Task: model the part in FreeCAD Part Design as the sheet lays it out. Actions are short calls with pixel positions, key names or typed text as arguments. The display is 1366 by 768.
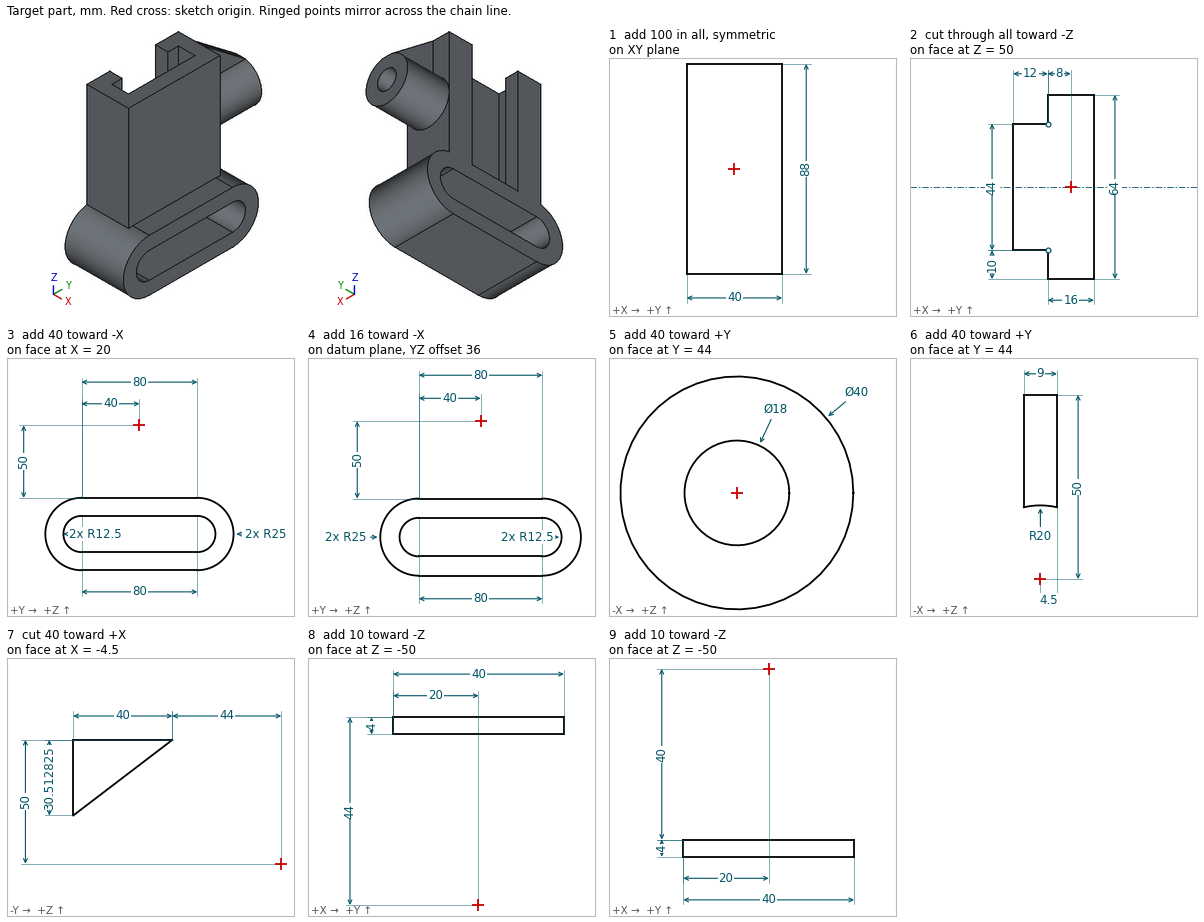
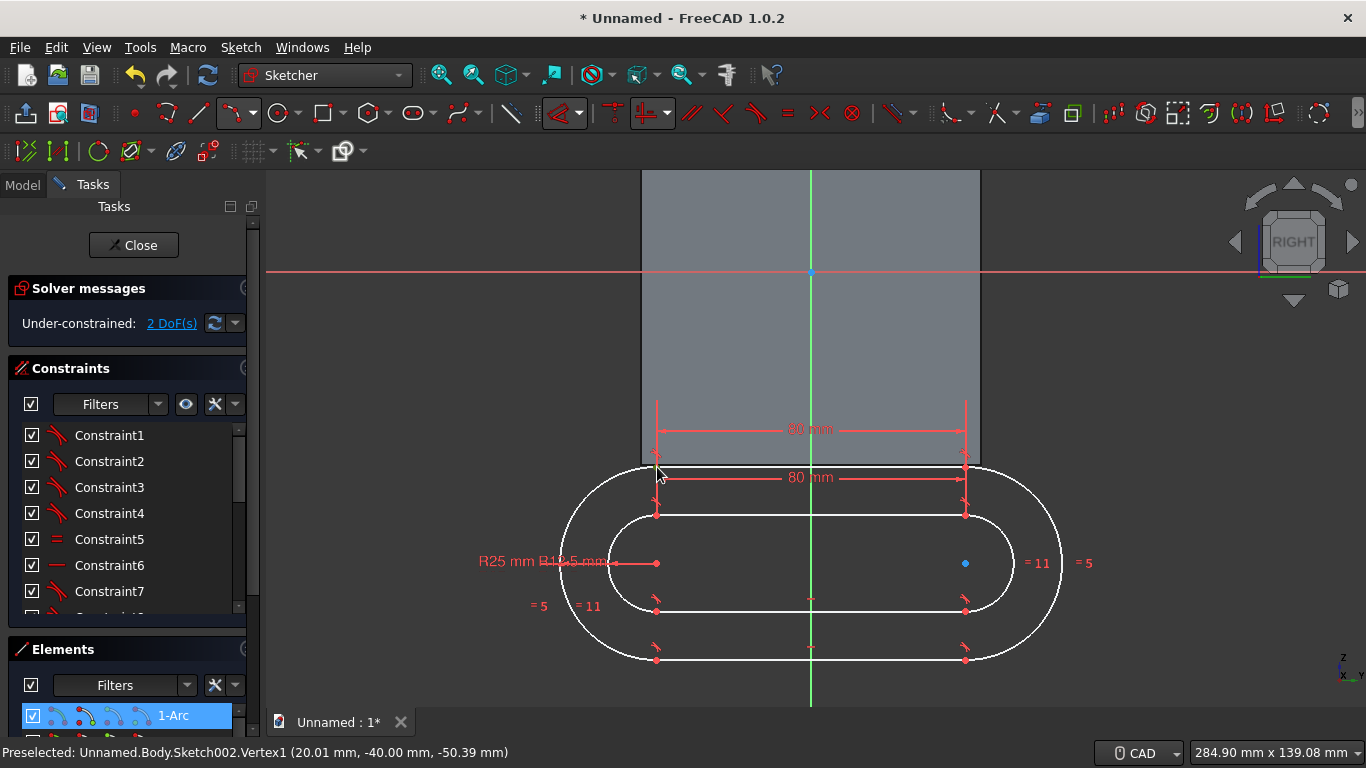
key(l)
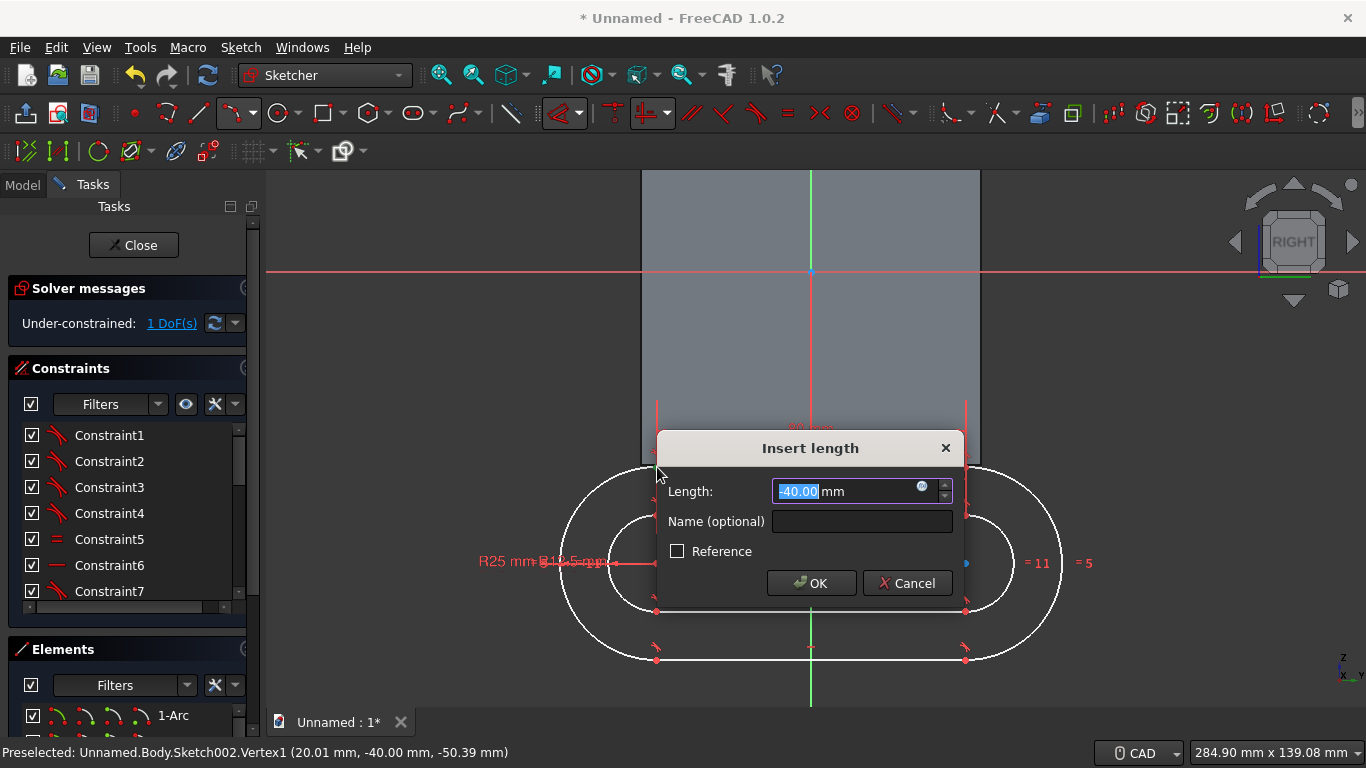
text(-40)
key(Return)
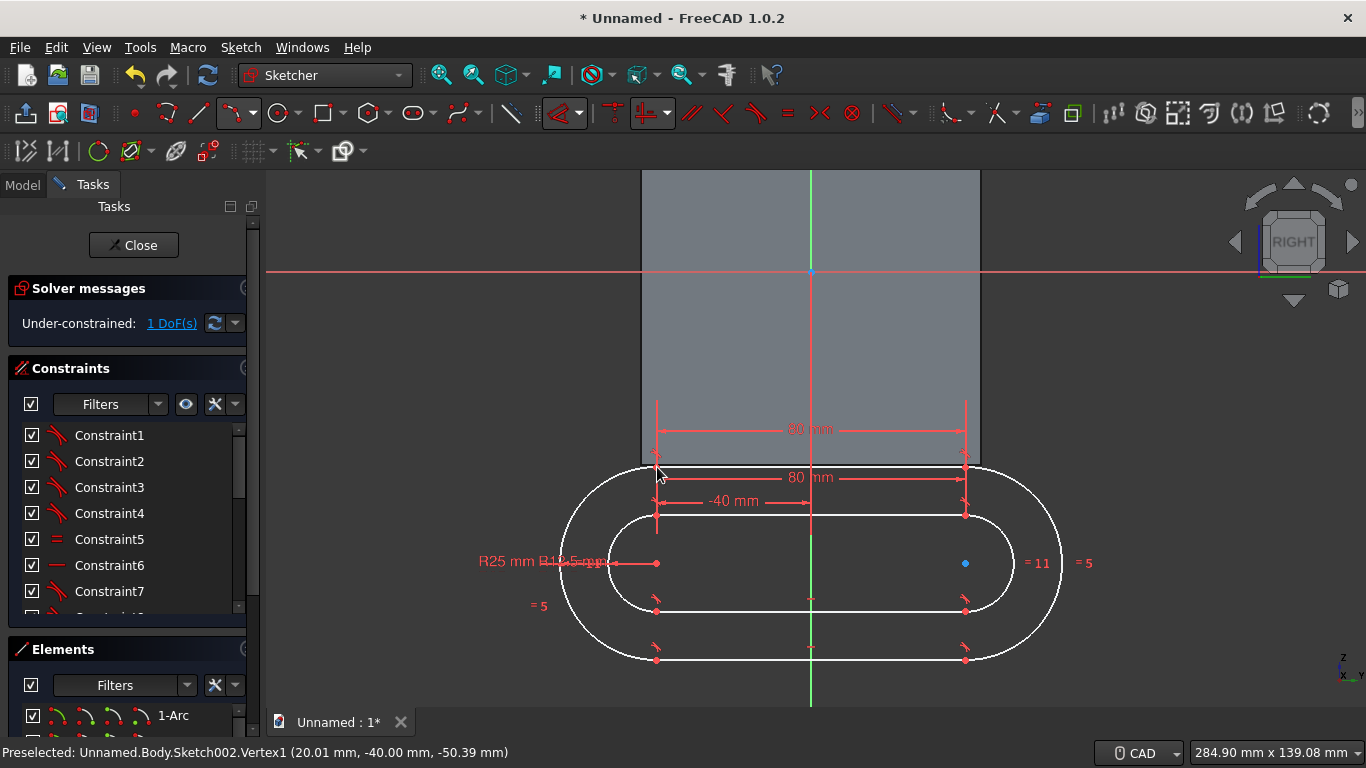
click(657, 467)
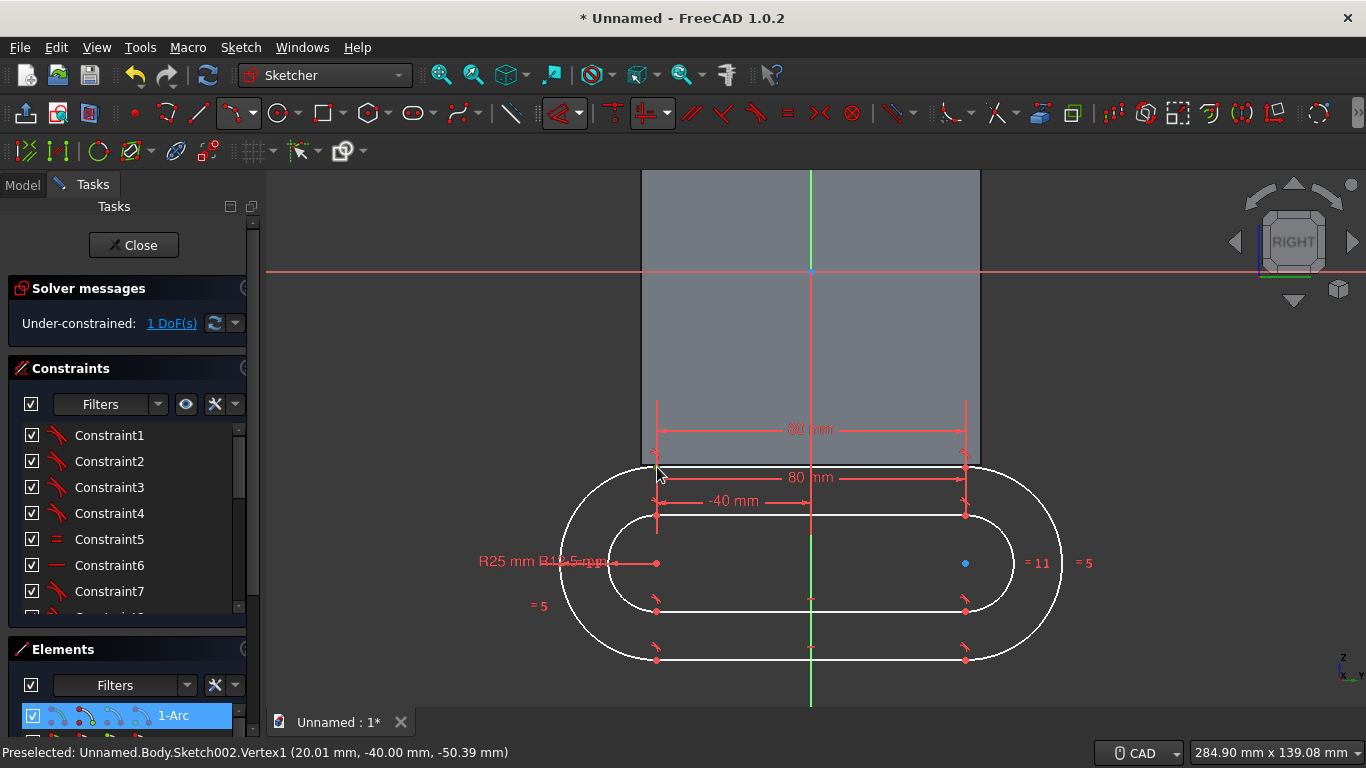
key(i)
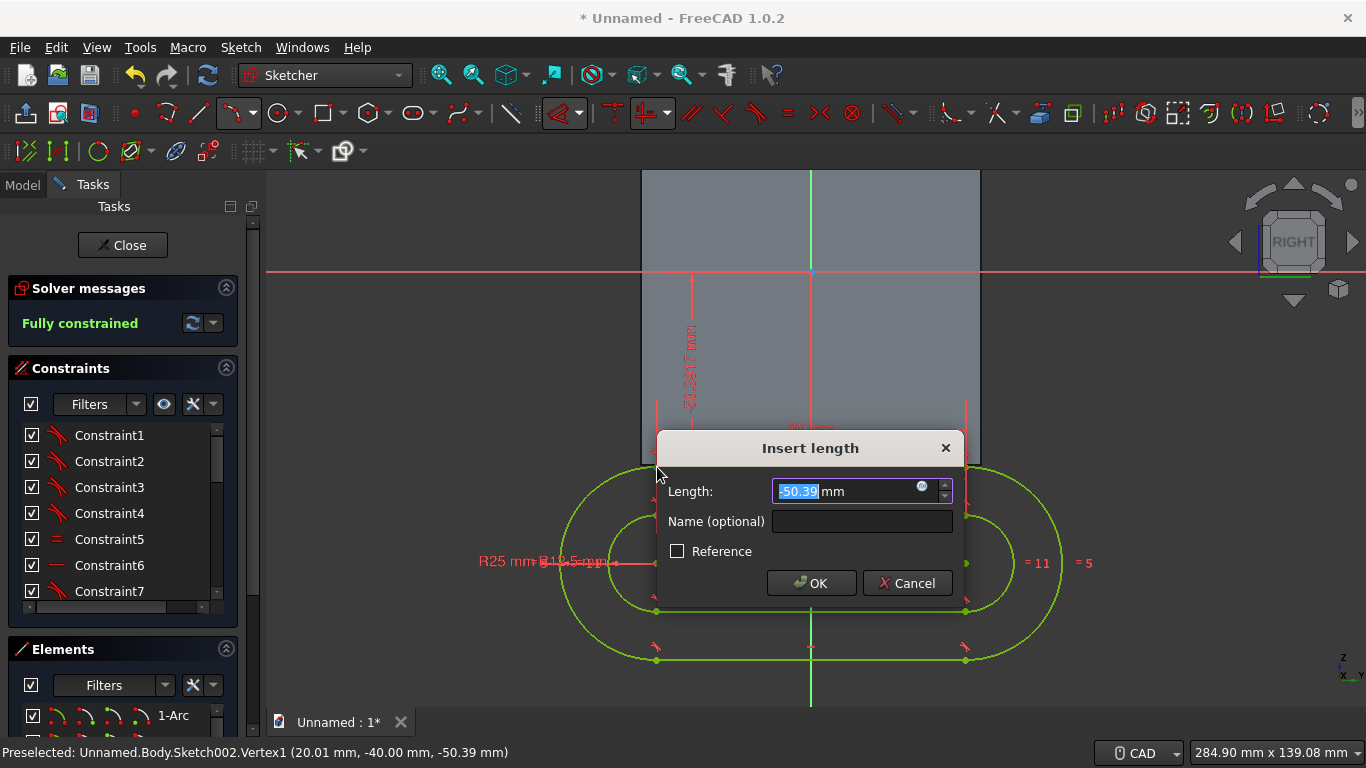
text(-50)
key(Return)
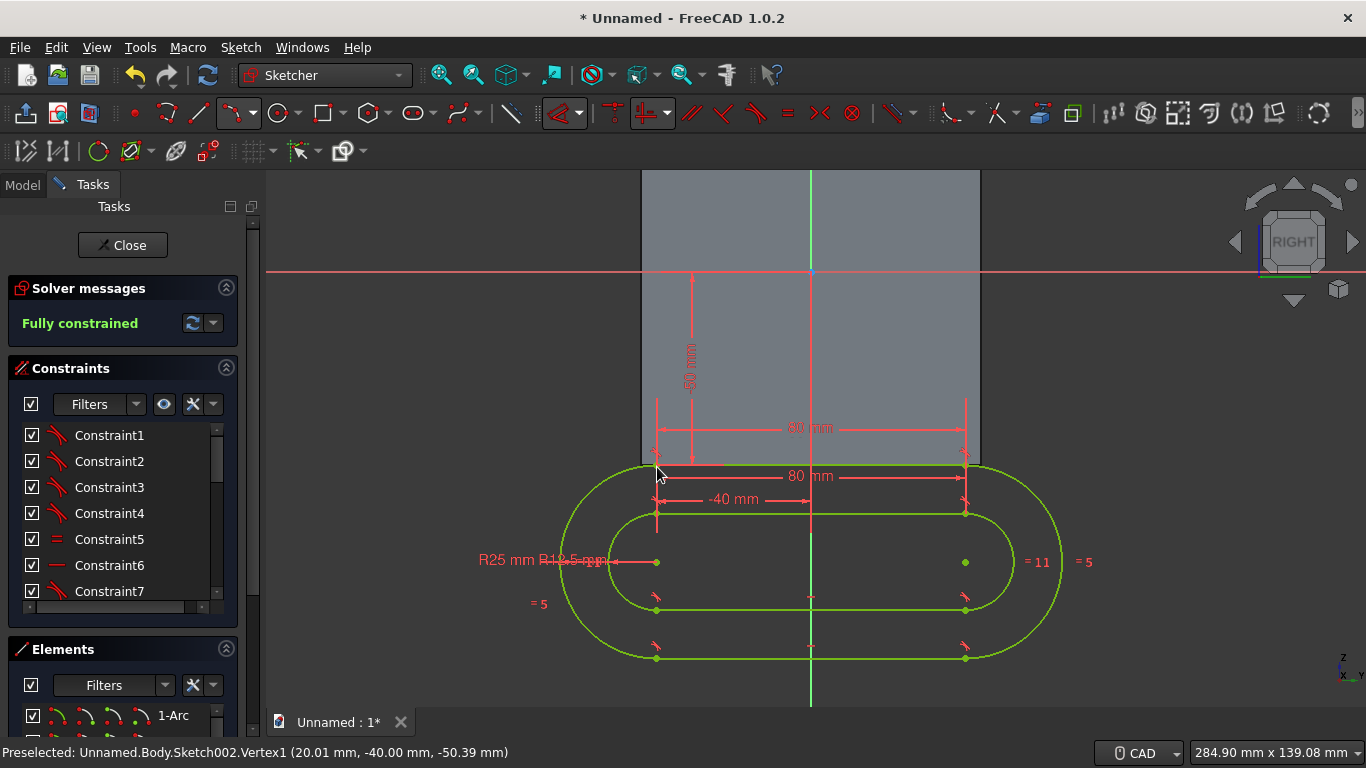
click(123, 245)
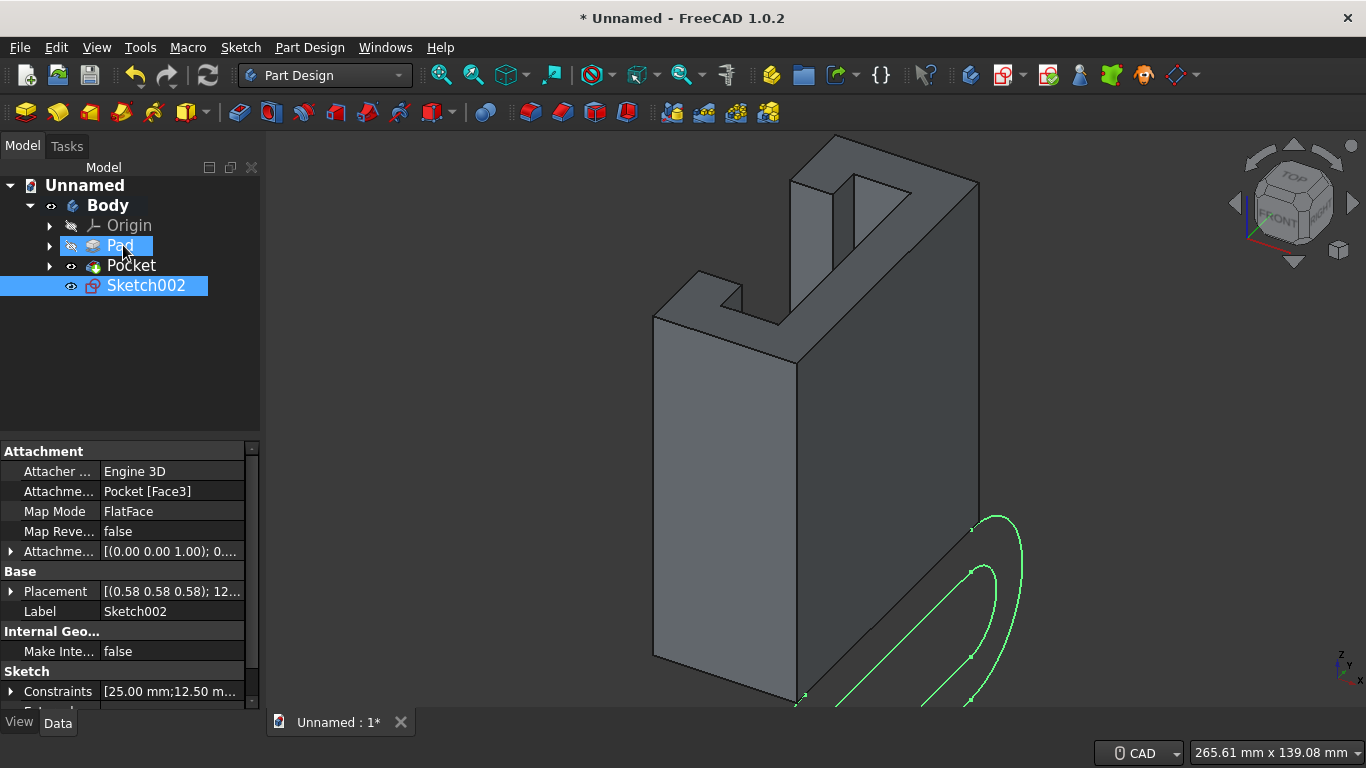
click(26, 112)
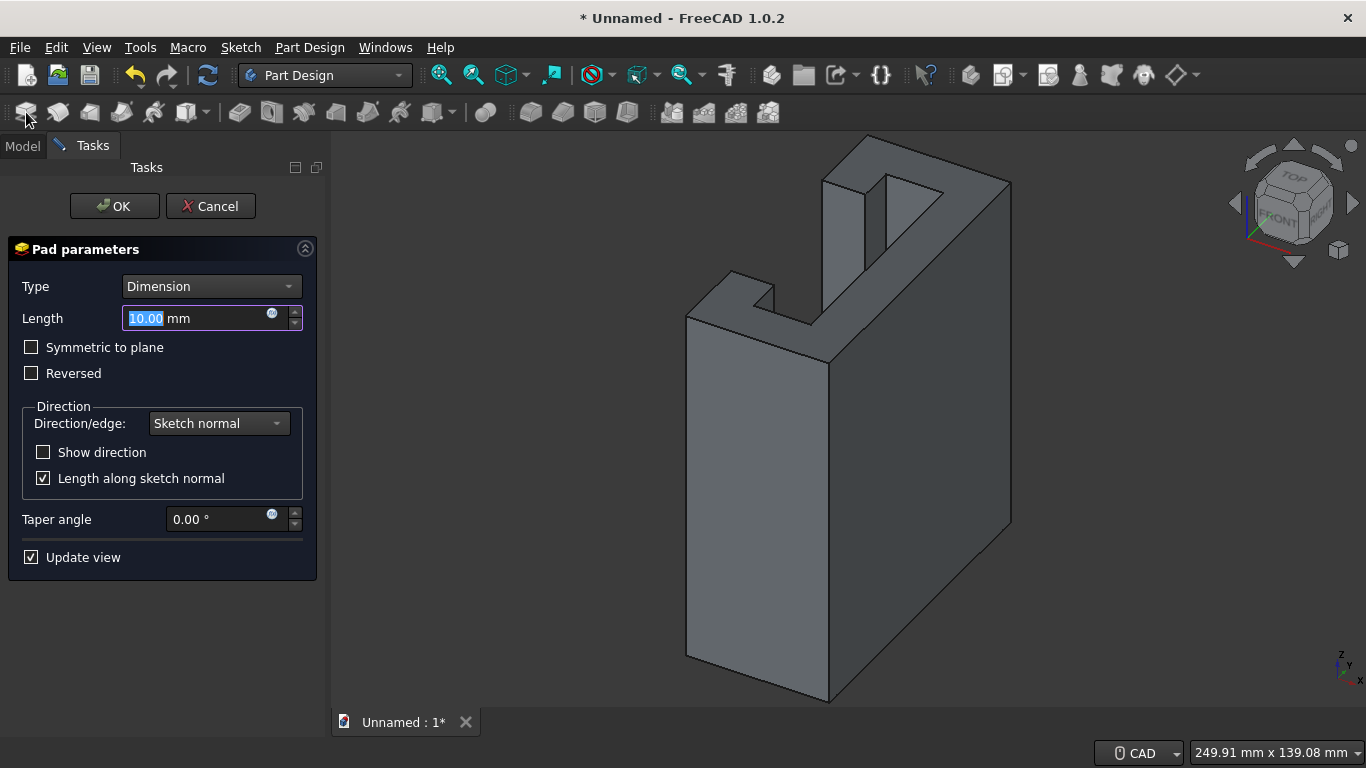
text(40)
key(Tab)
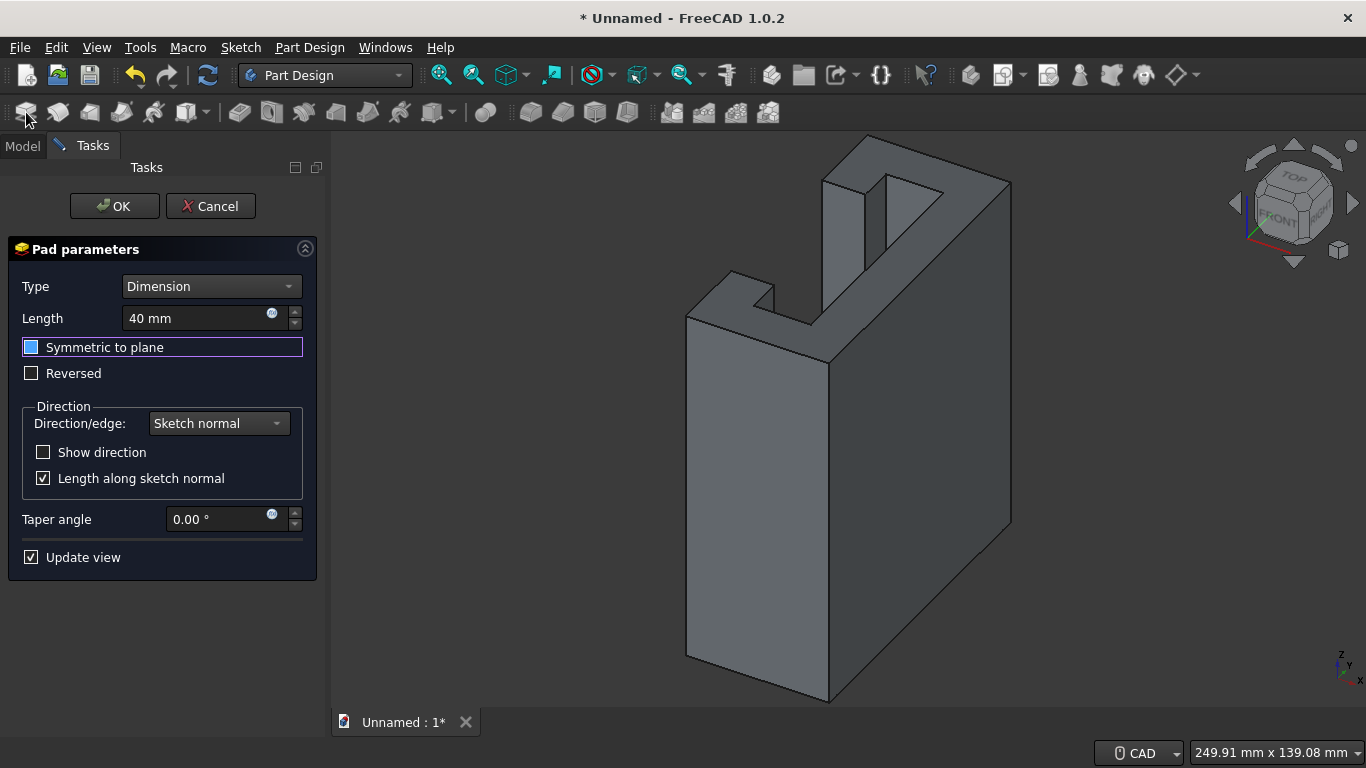
click(30, 373)